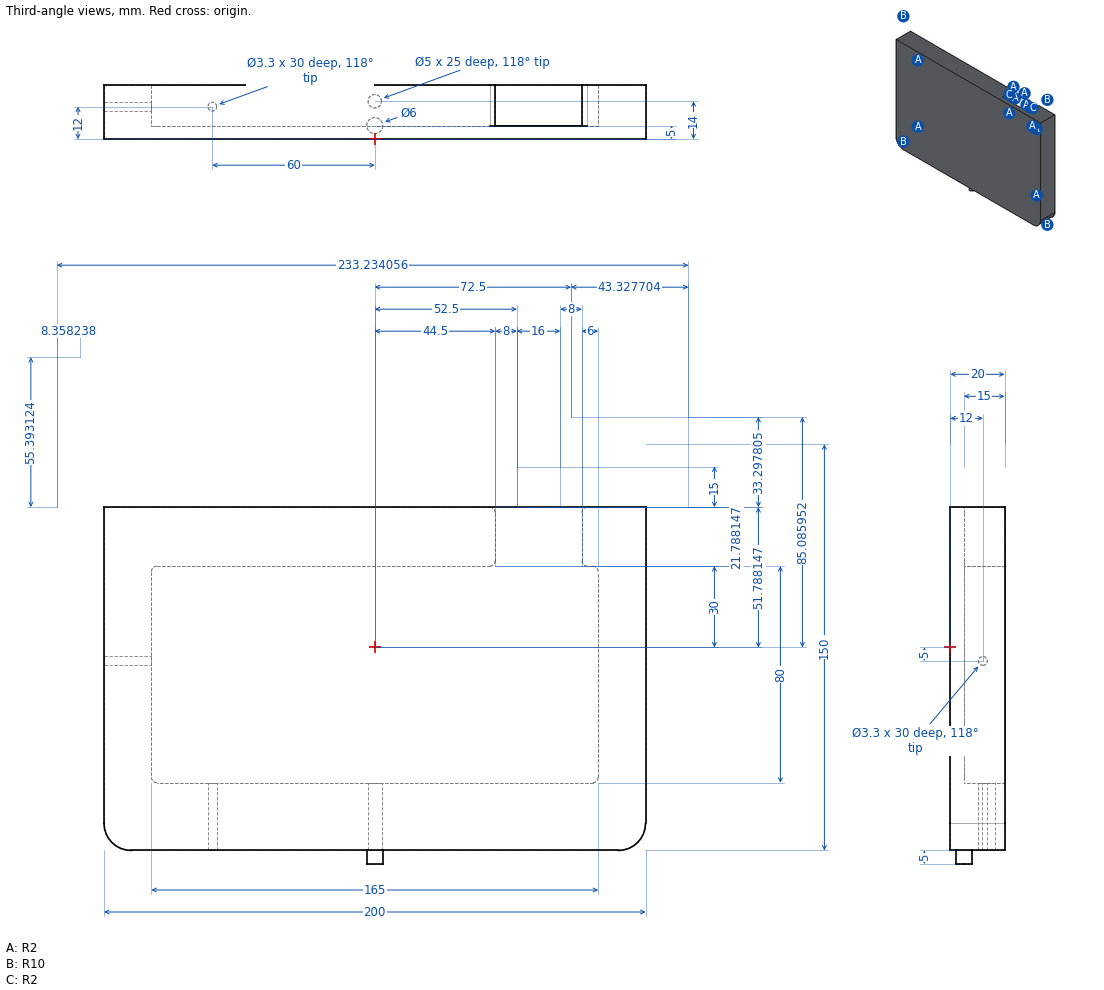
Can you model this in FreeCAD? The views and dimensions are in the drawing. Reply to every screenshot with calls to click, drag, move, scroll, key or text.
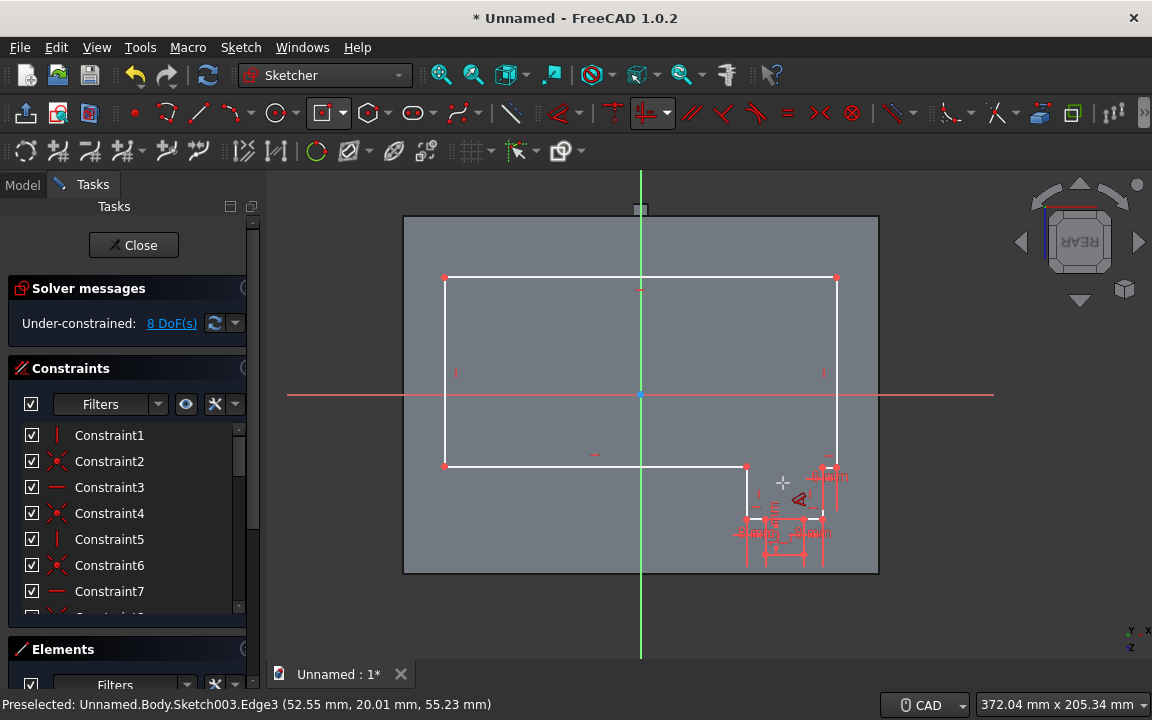
click(777, 555)
click(785, 589)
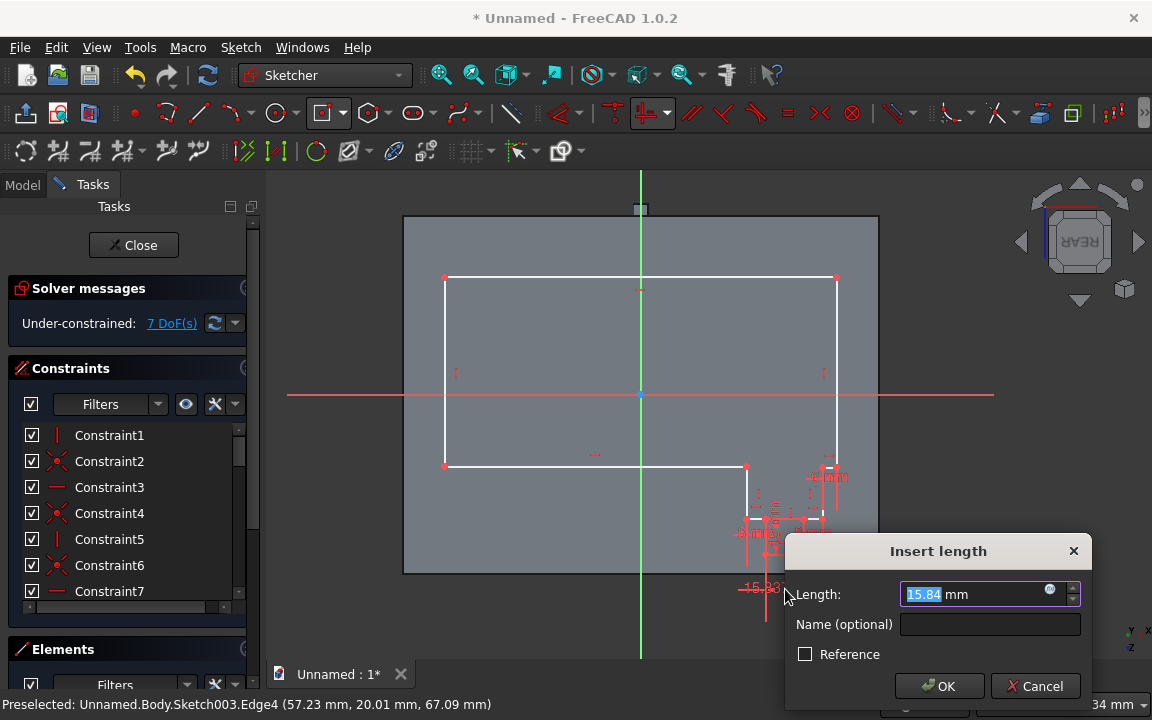
text(16)
key(Return)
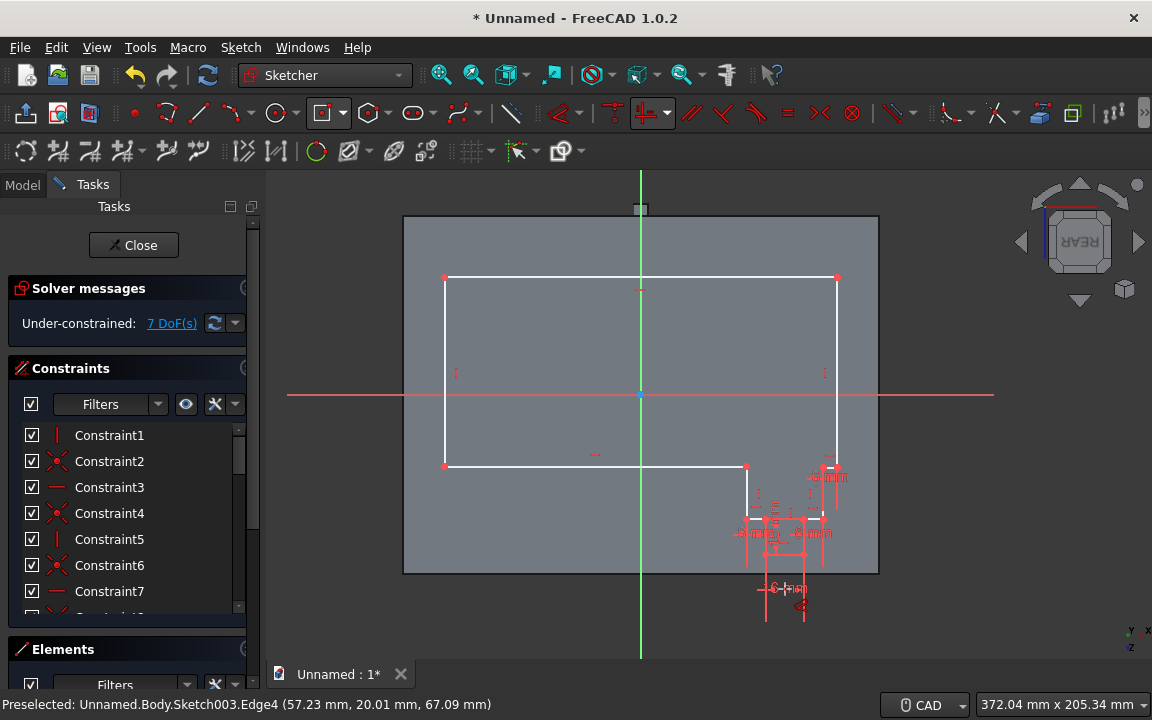
scroll(804, 544, up, 2)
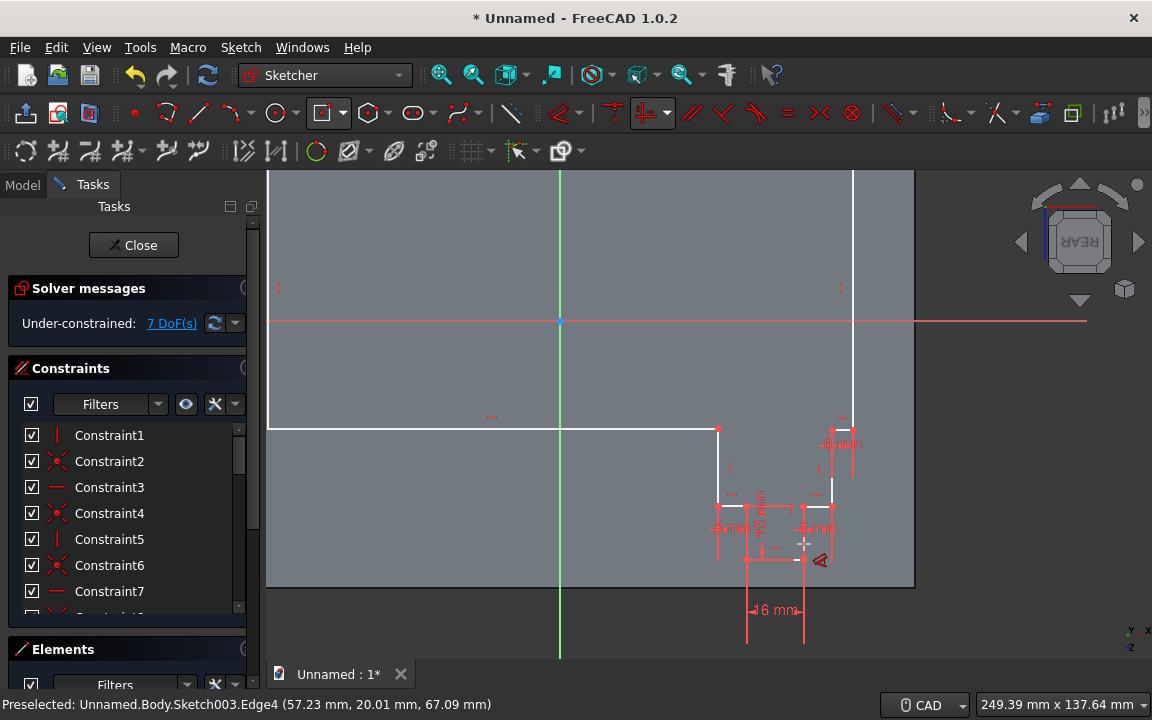
click(804, 544)
click(838, 552)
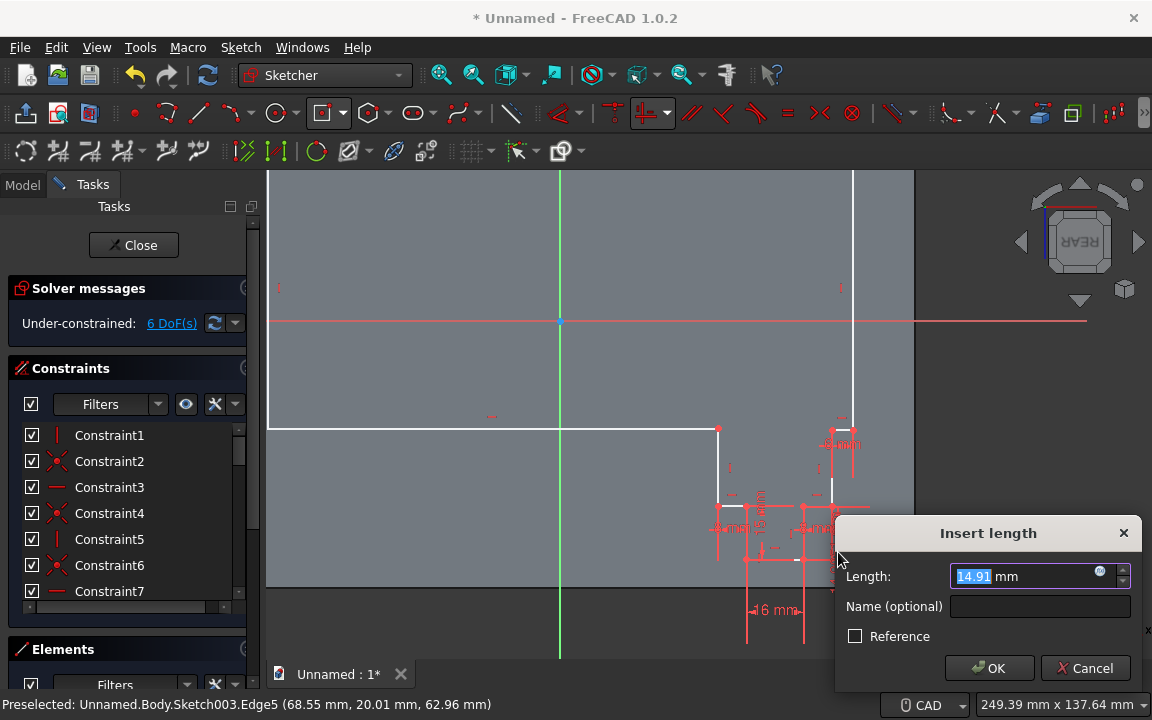
text(15)
key(Return)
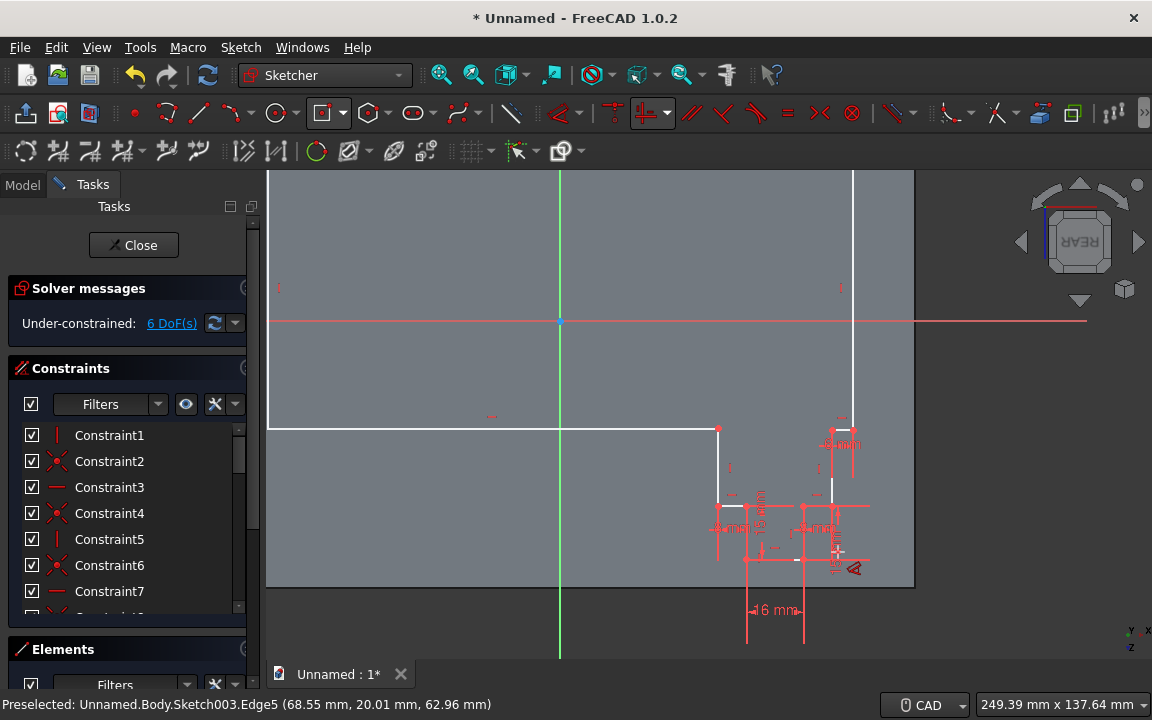
click(853, 345)
click(887, 261)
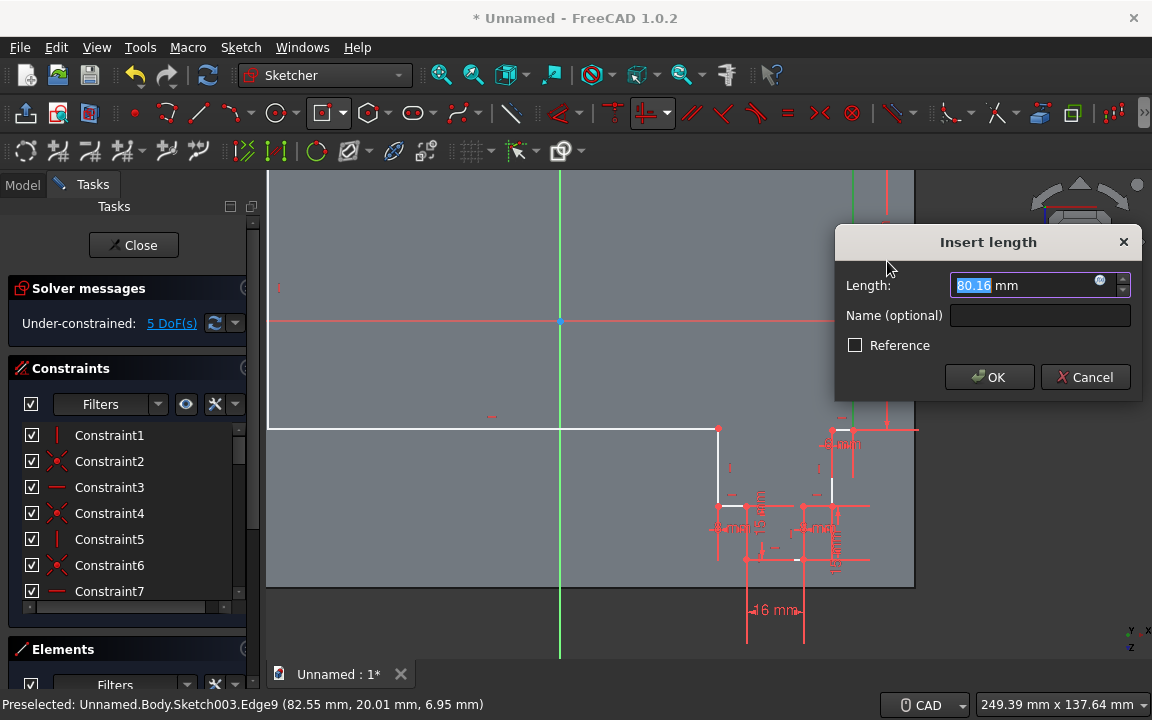
text(80)
key(Return)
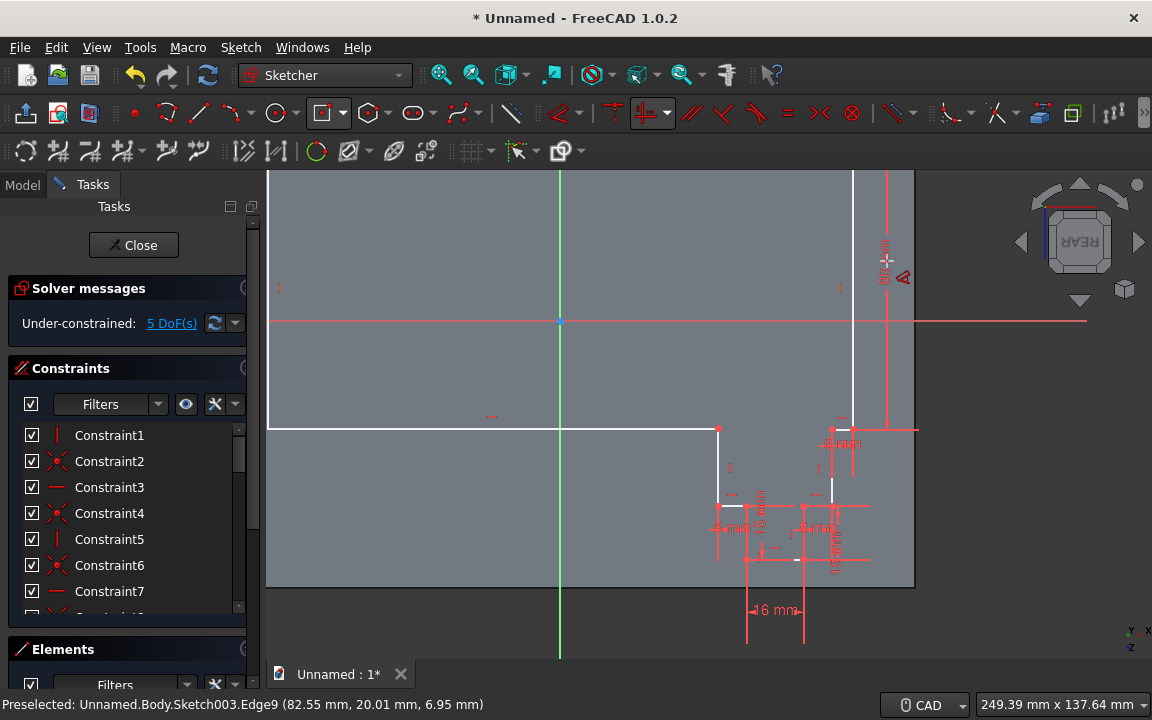
scroll(804, 543, down, 2)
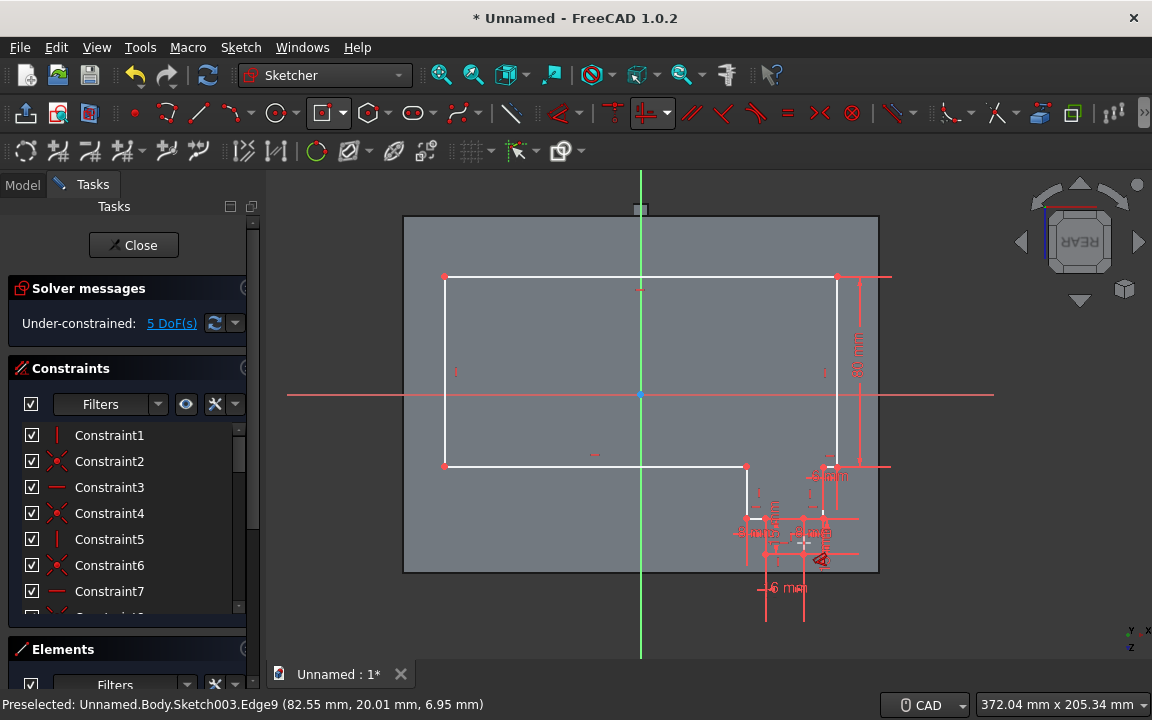
click(445, 334)
click(411, 372)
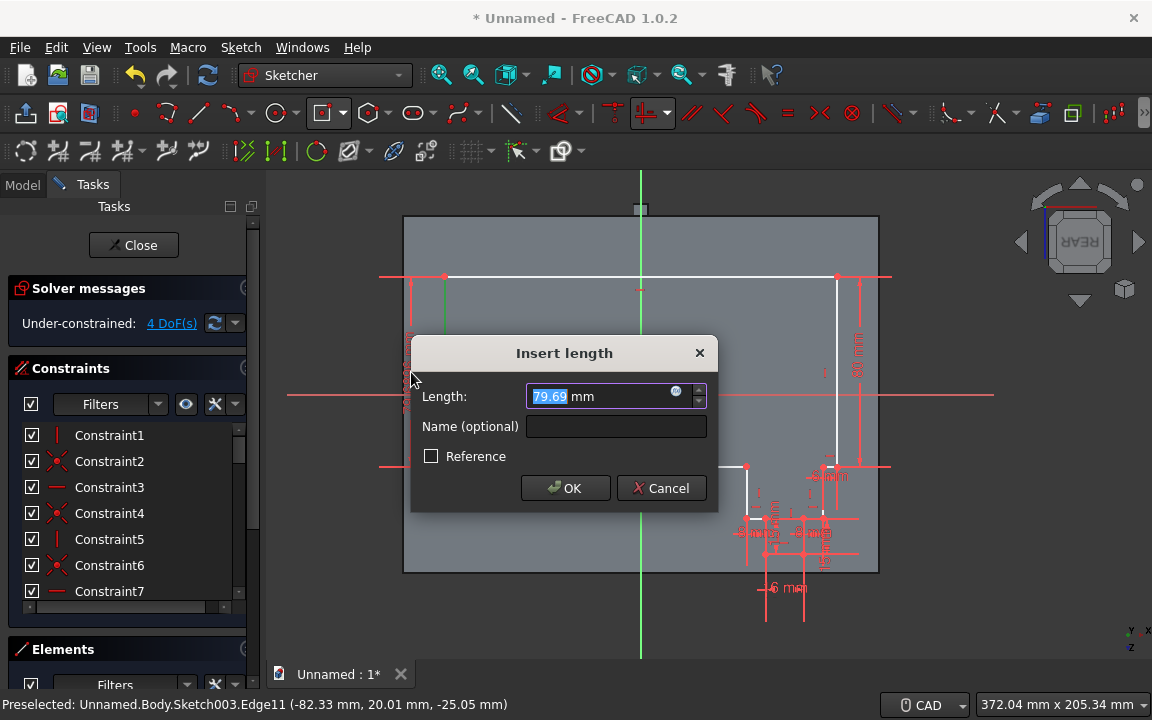
text(80)
key(Return)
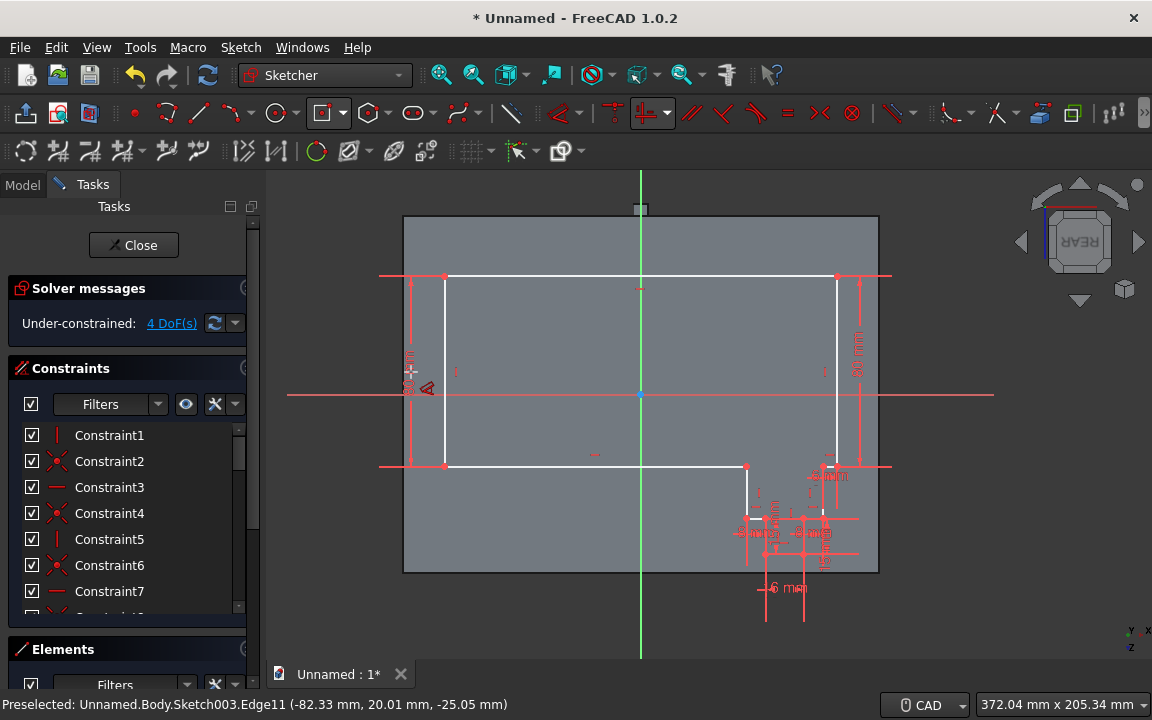
click(720, 276)
click(551, 242)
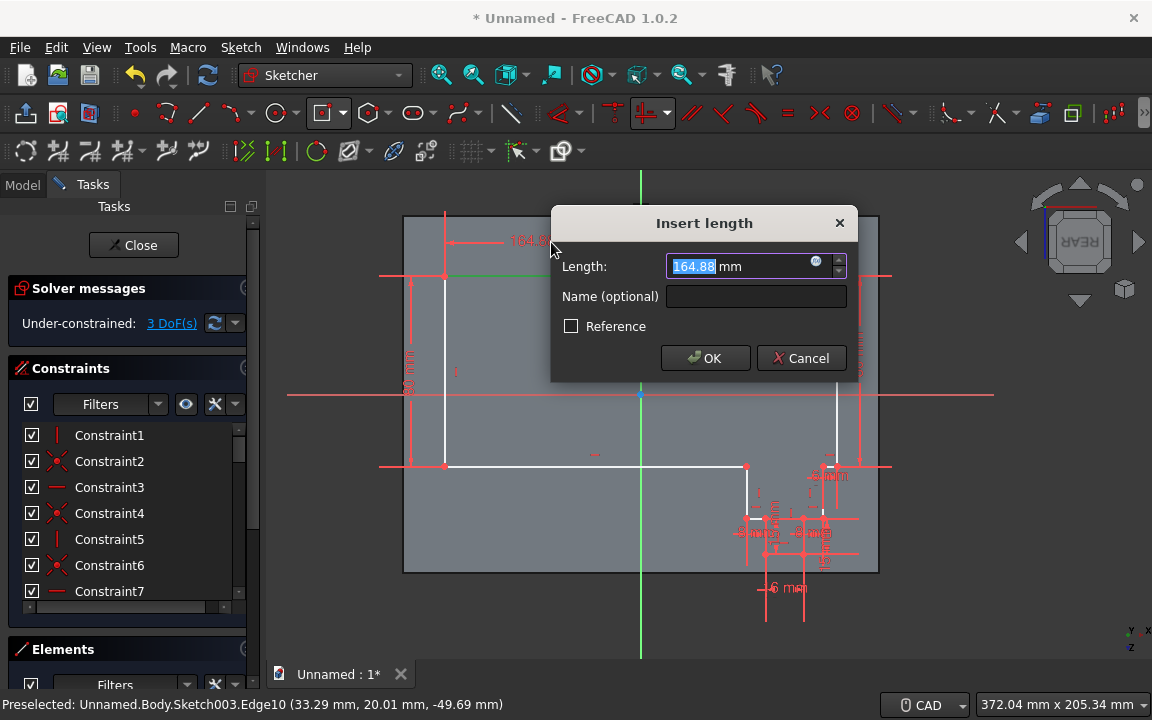
text(165)
key(Return)